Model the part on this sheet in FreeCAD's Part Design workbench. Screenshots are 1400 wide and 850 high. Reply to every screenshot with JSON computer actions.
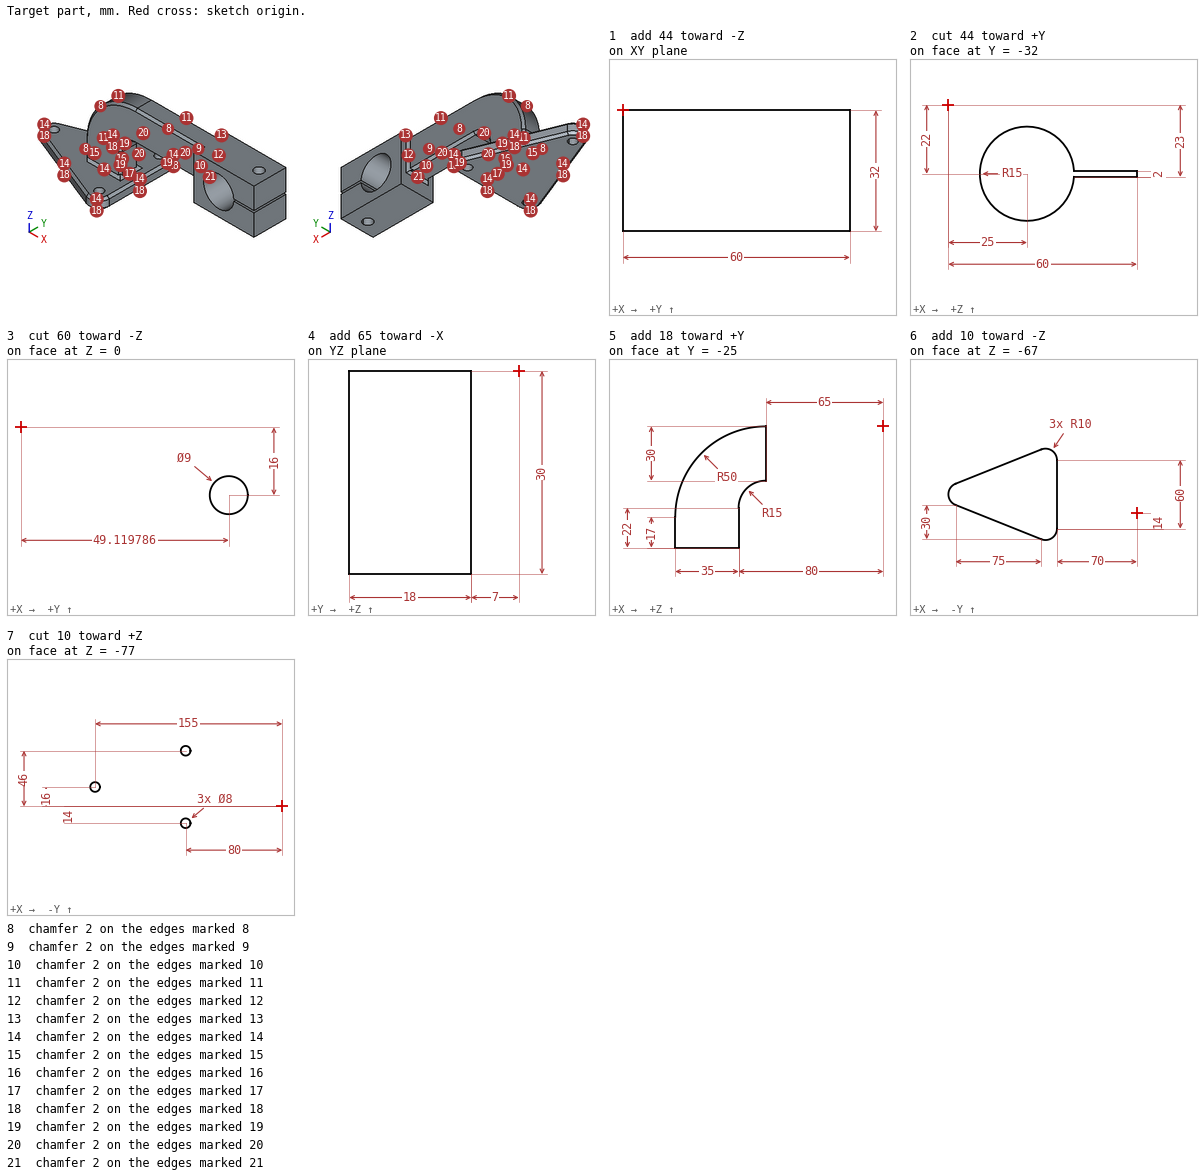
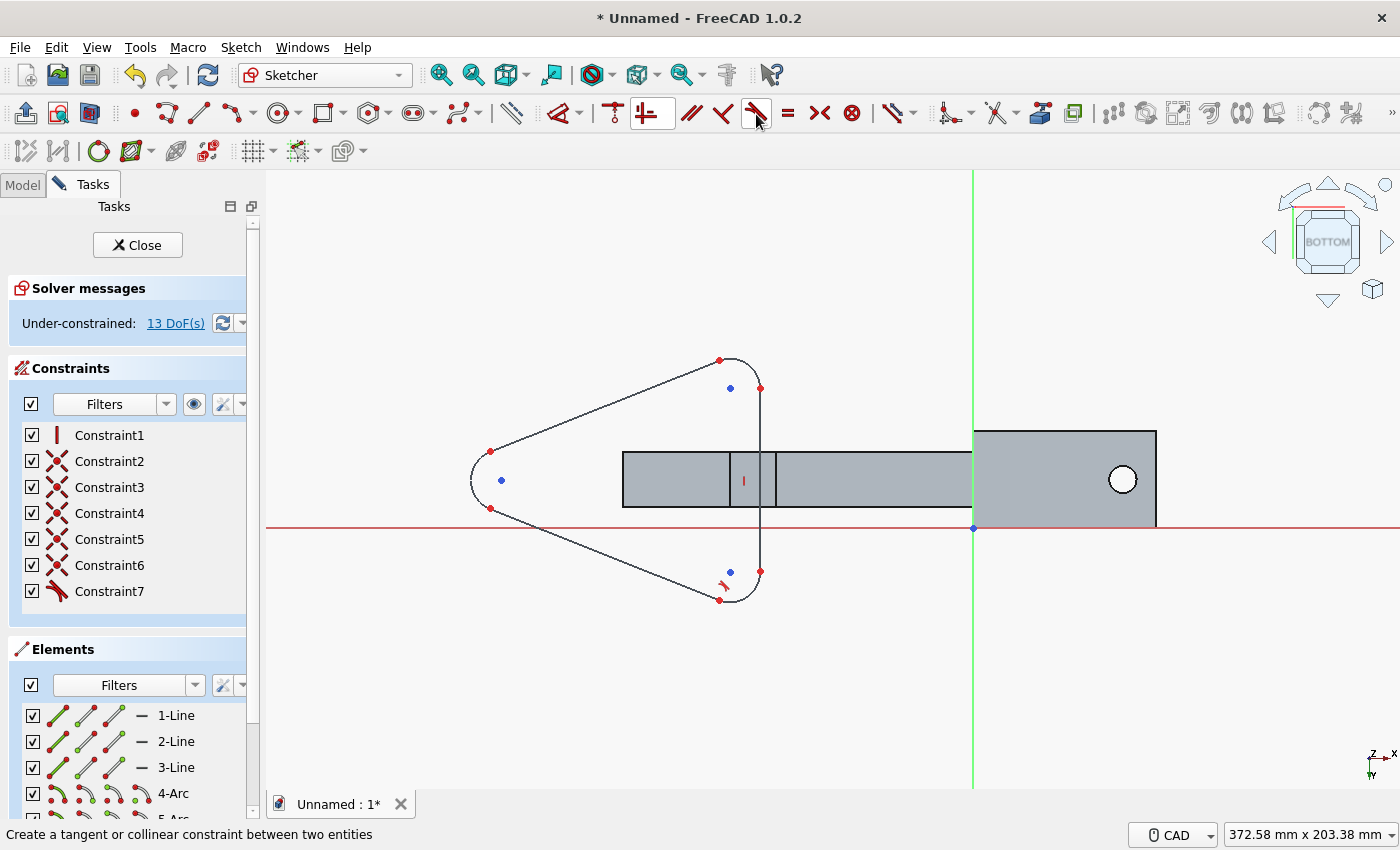
{"action": "left_click", "coordinate": [650, 573]}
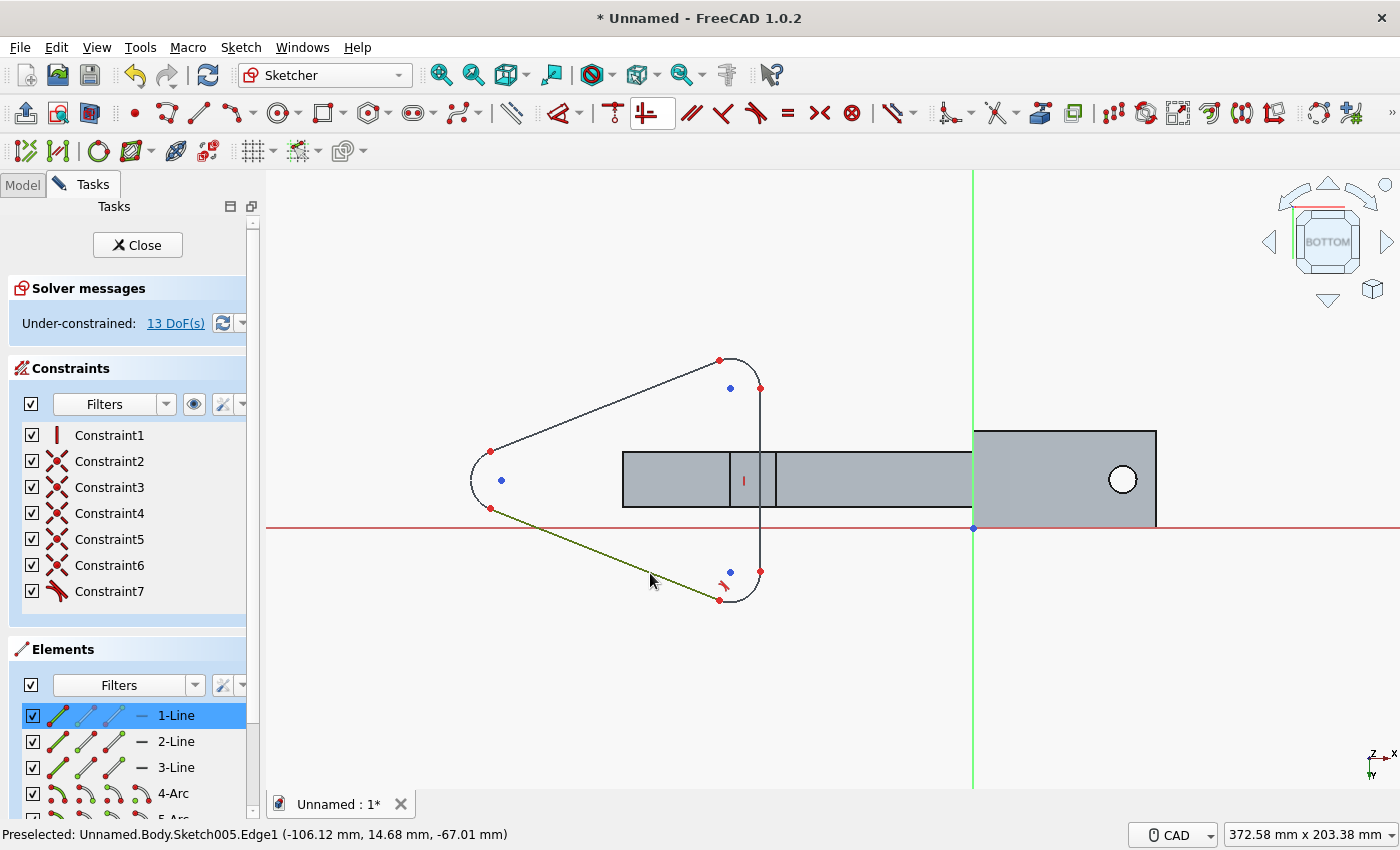
{"action": "left_click", "coordinate": [474, 467]}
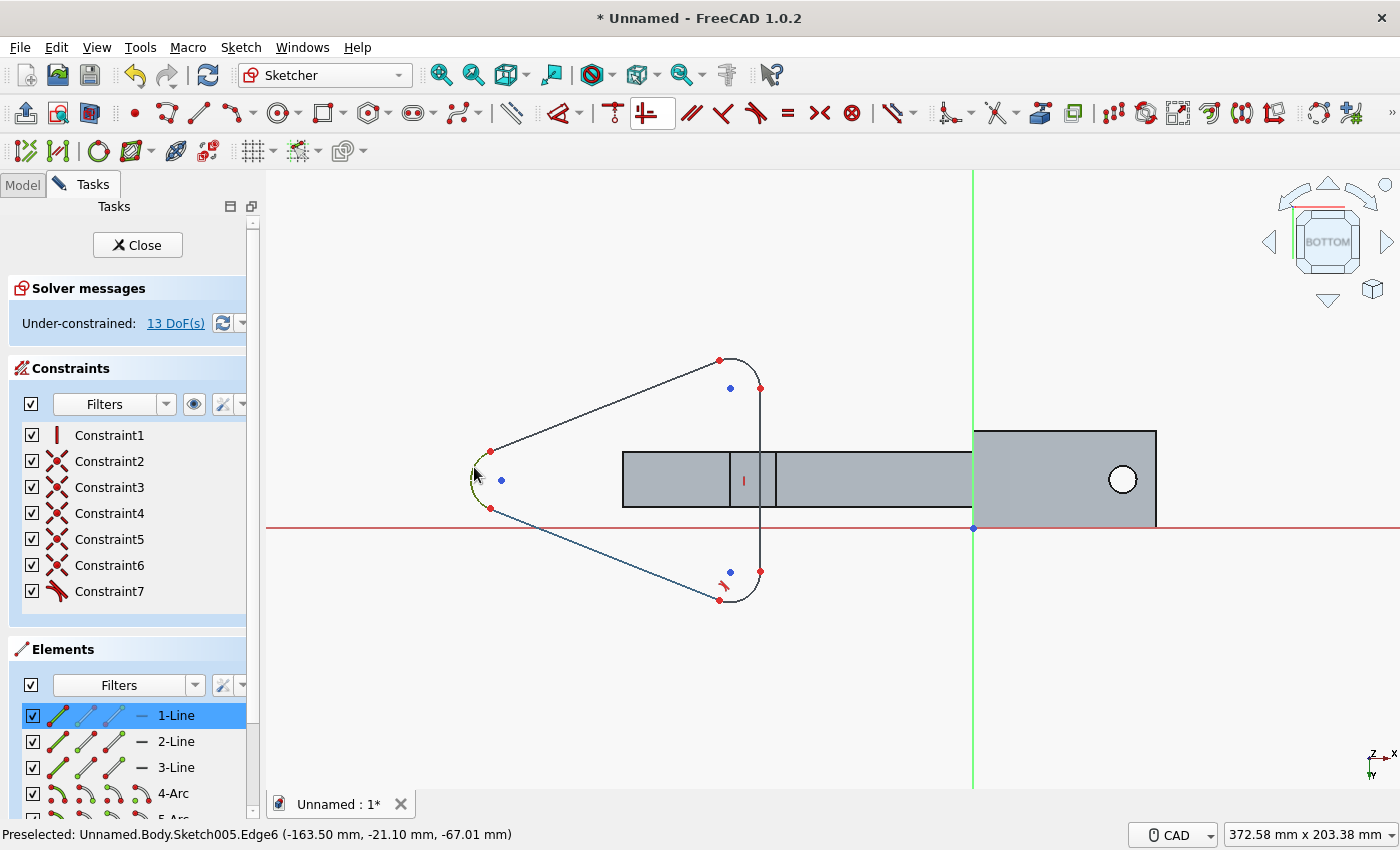
{"action": "left_click", "coordinate": [756, 114]}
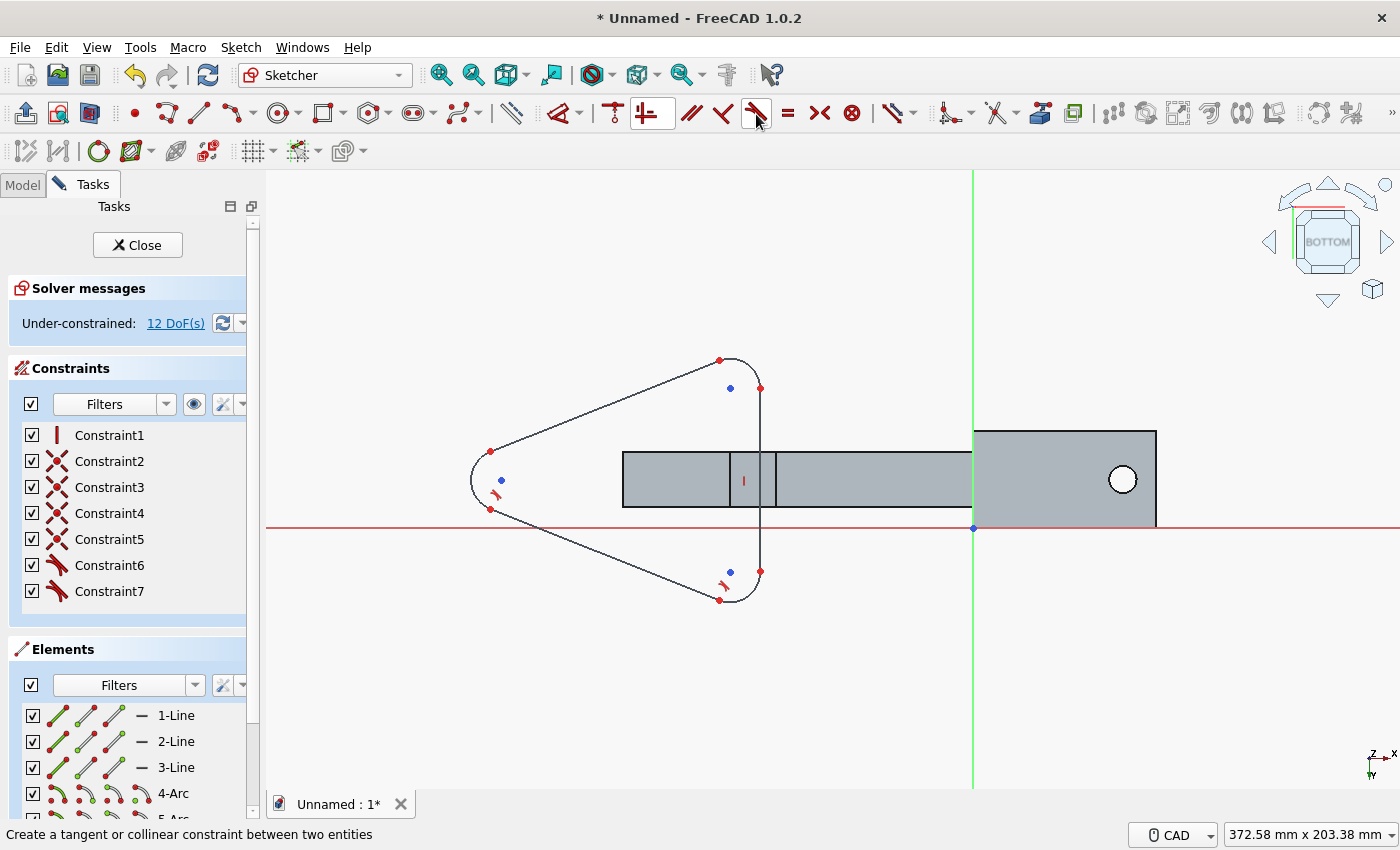
{"action": "scroll", "coordinate": [760, 517], "scroll_direction": "up", "scroll_amount": 2}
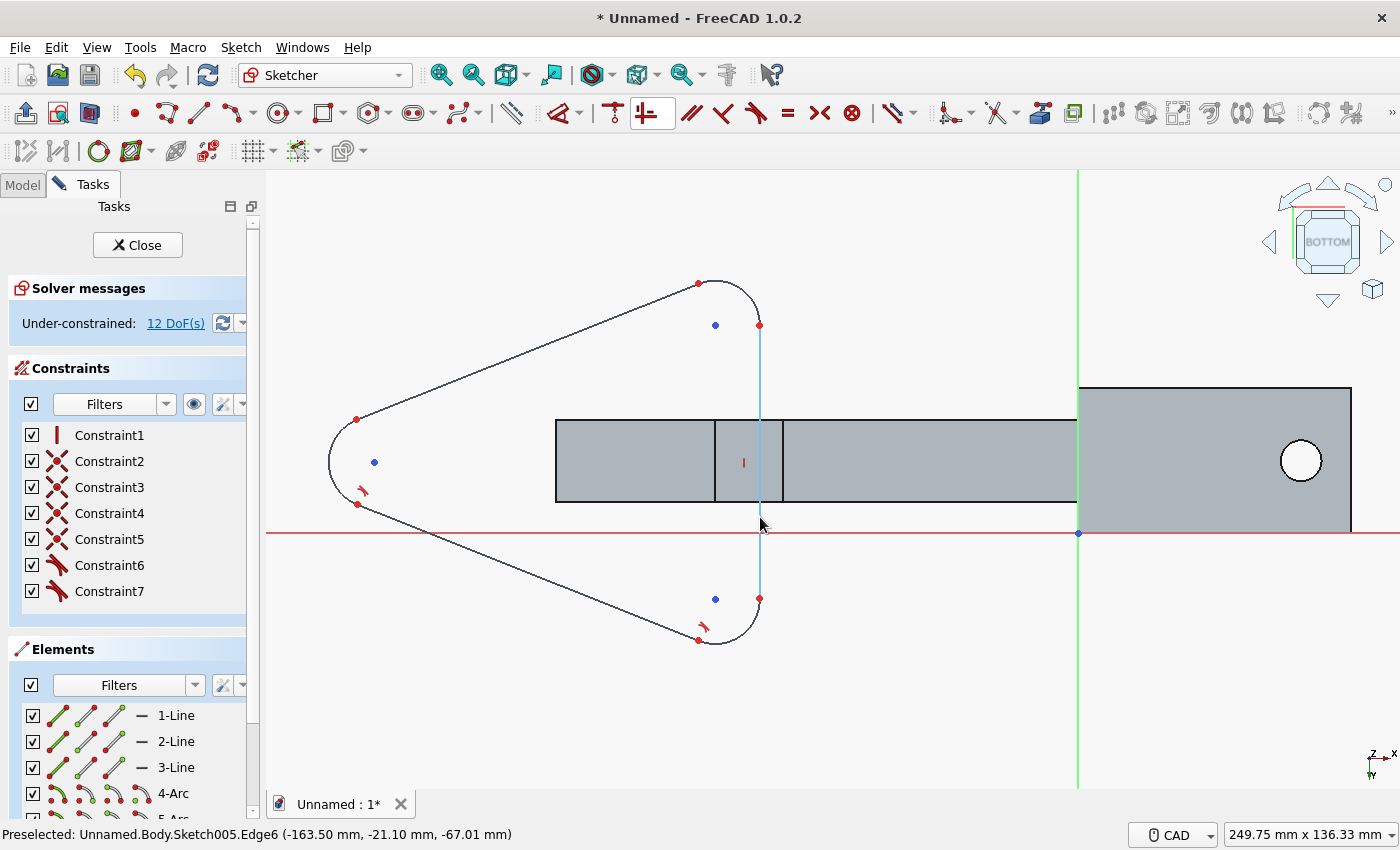
{"action": "left_click", "coordinate": [760, 517]}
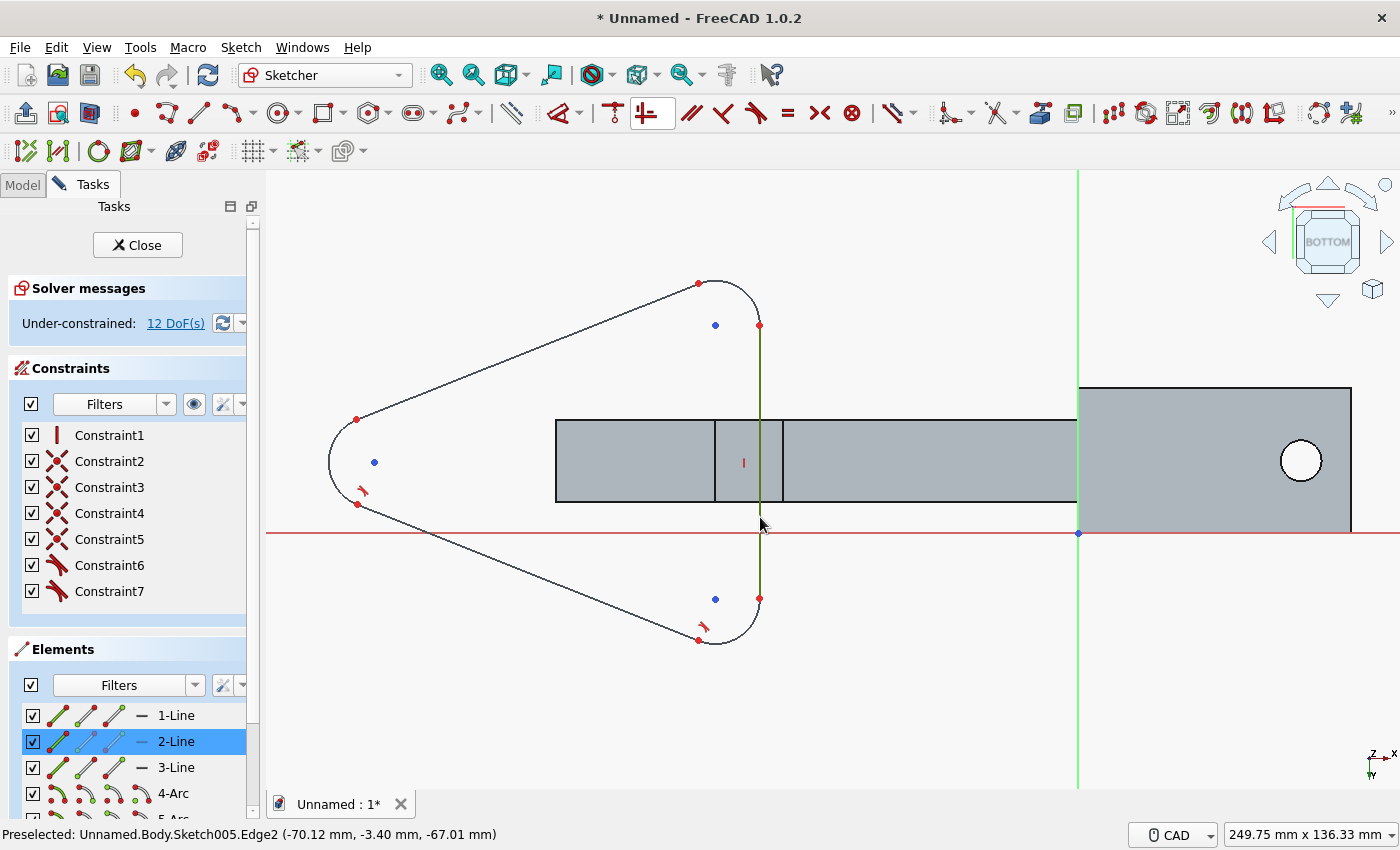
{"action": "left_click", "coordinate": [724, 643]}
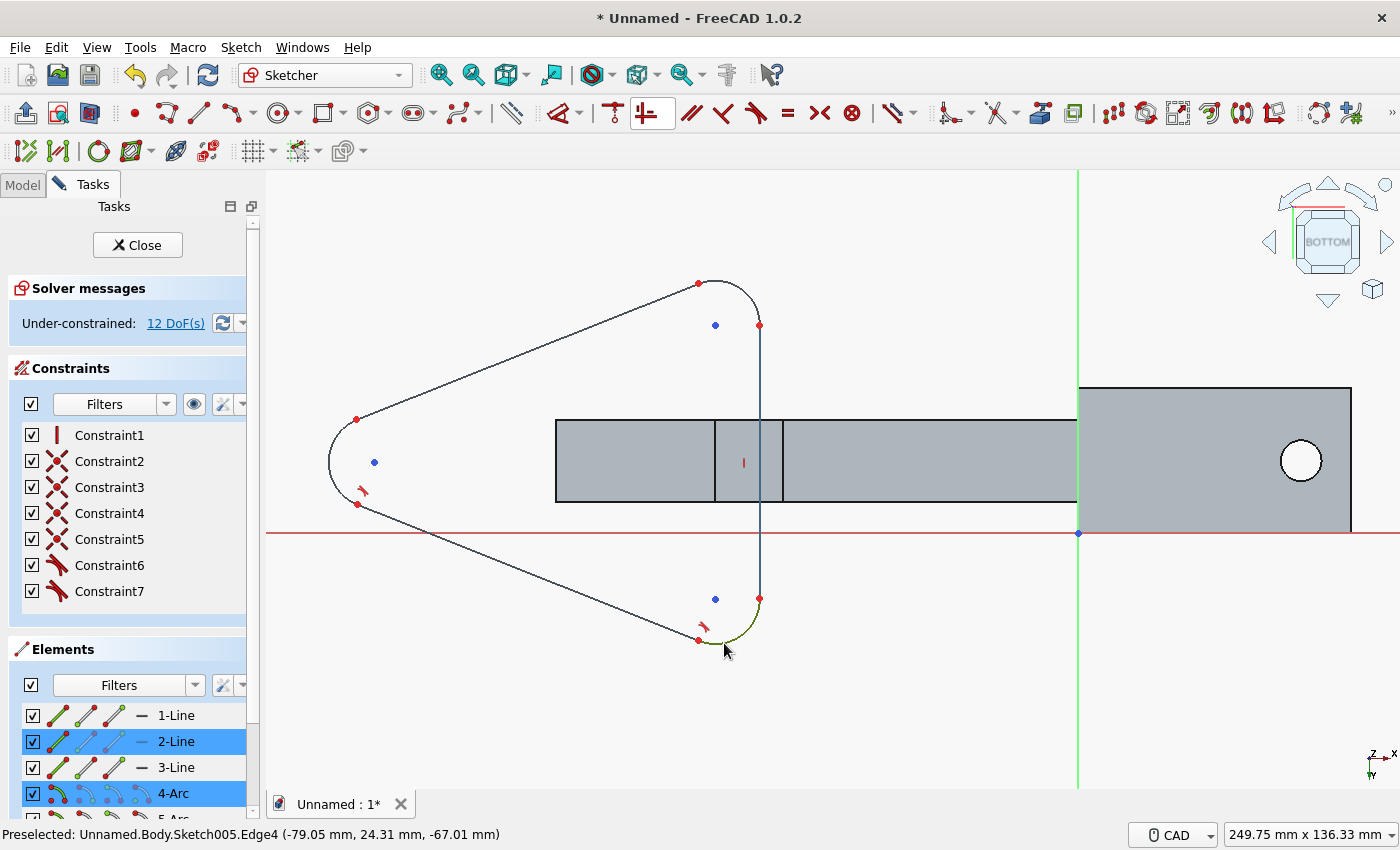
{"action": "left_click", "coordinate": [756, 114]}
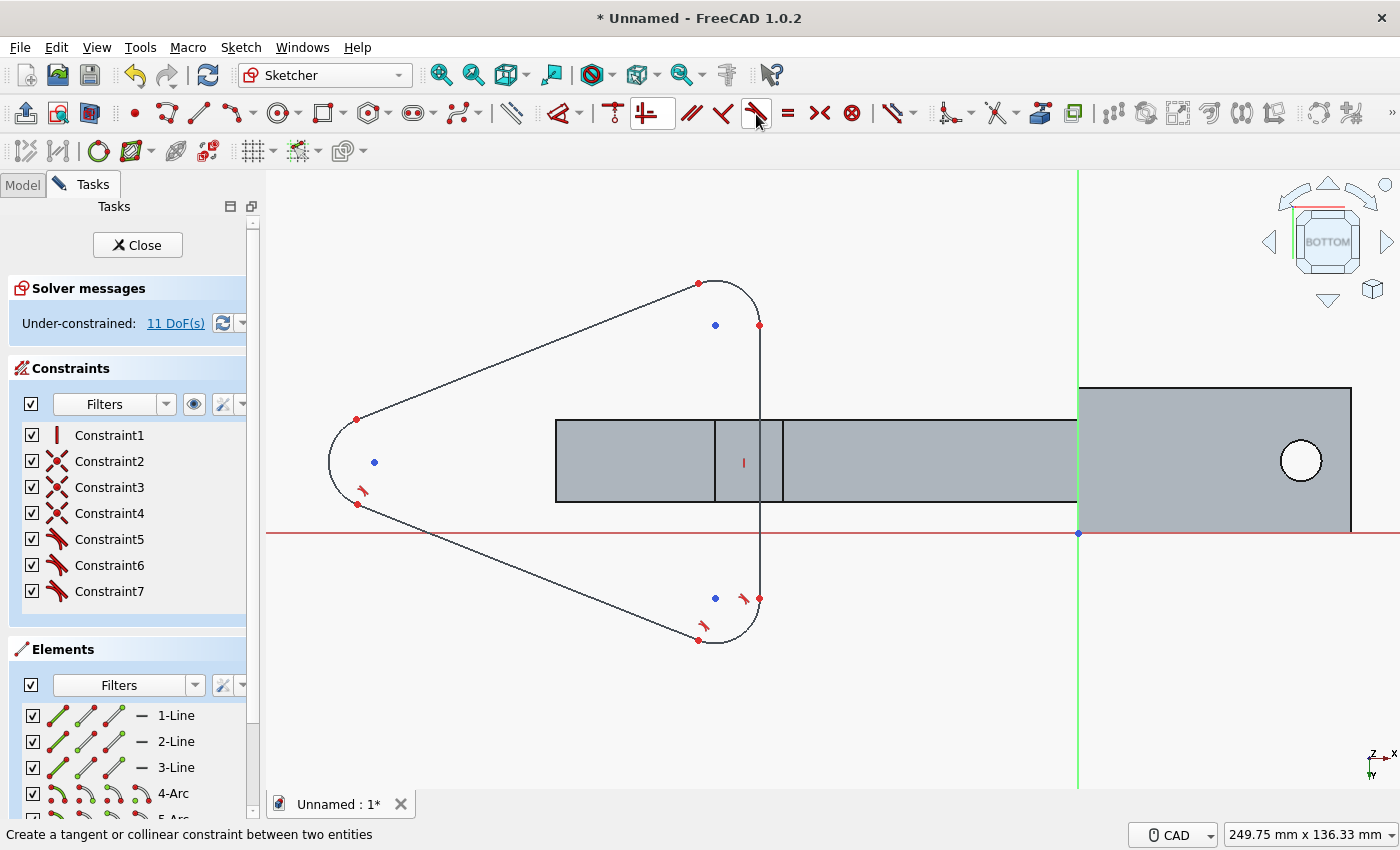
{"action": "left_click", "coordinate": [760, 517]}